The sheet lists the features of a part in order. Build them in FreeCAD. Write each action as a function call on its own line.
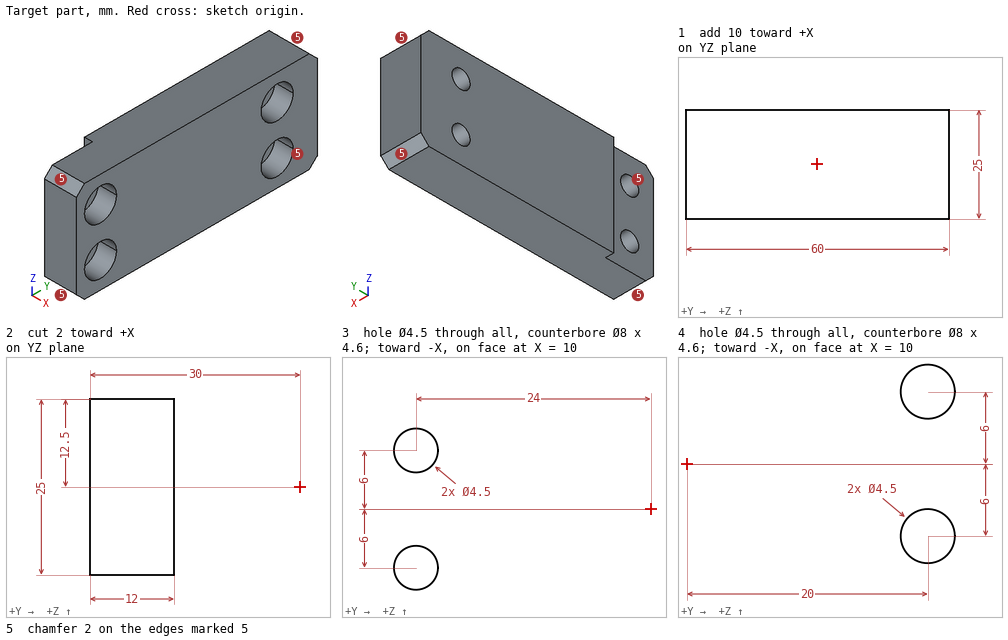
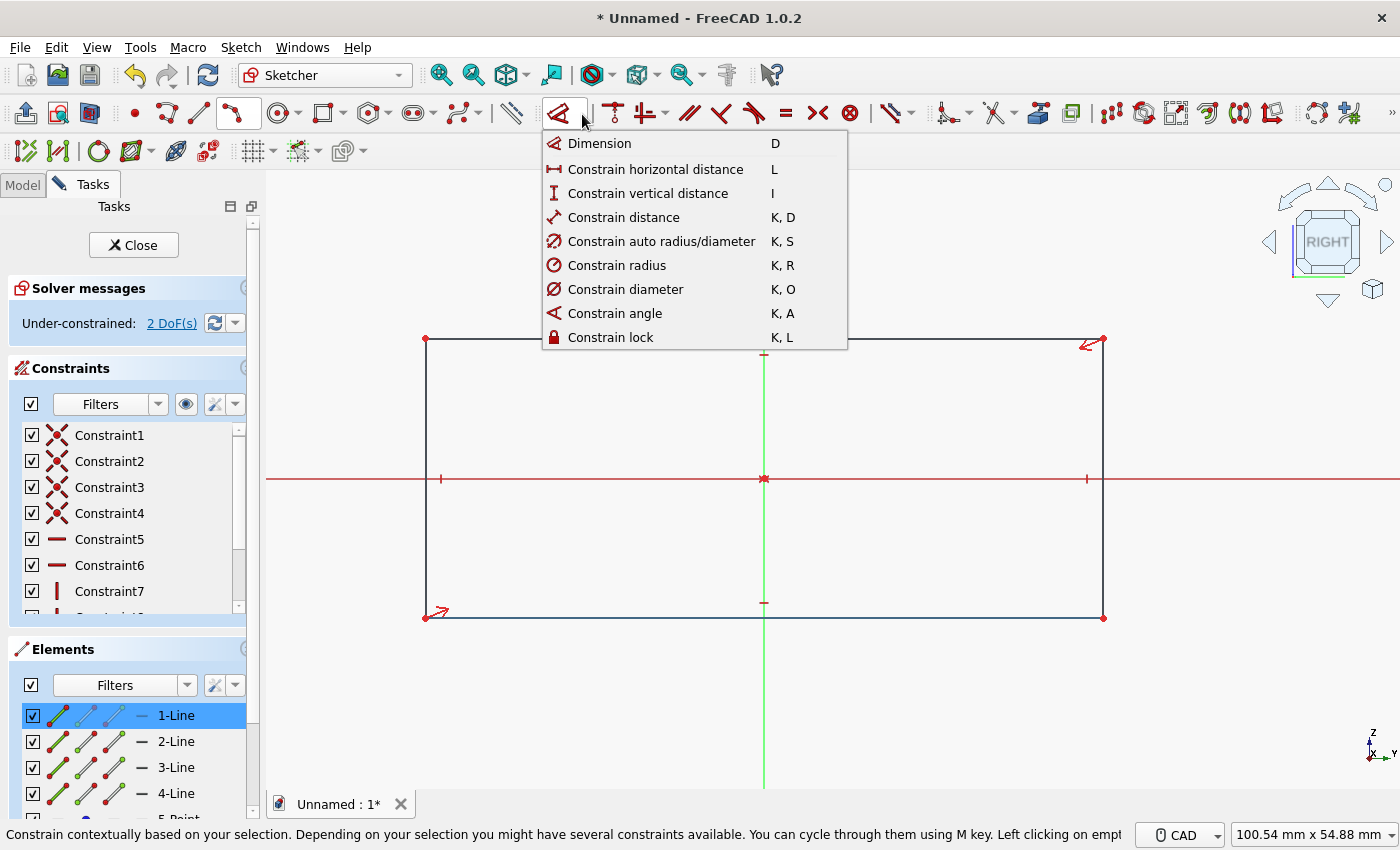
click(695, 169)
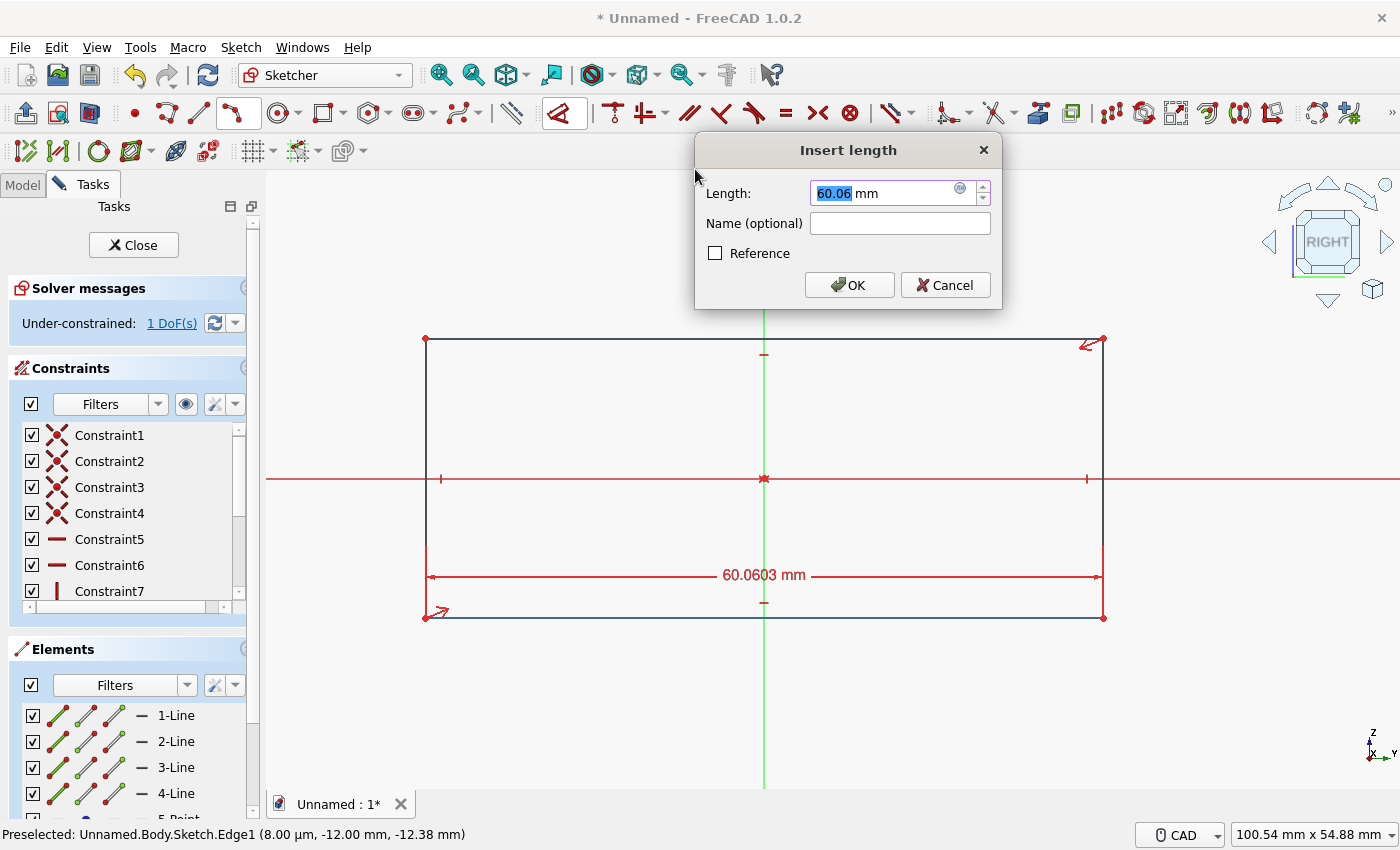
text(60)
key(Return)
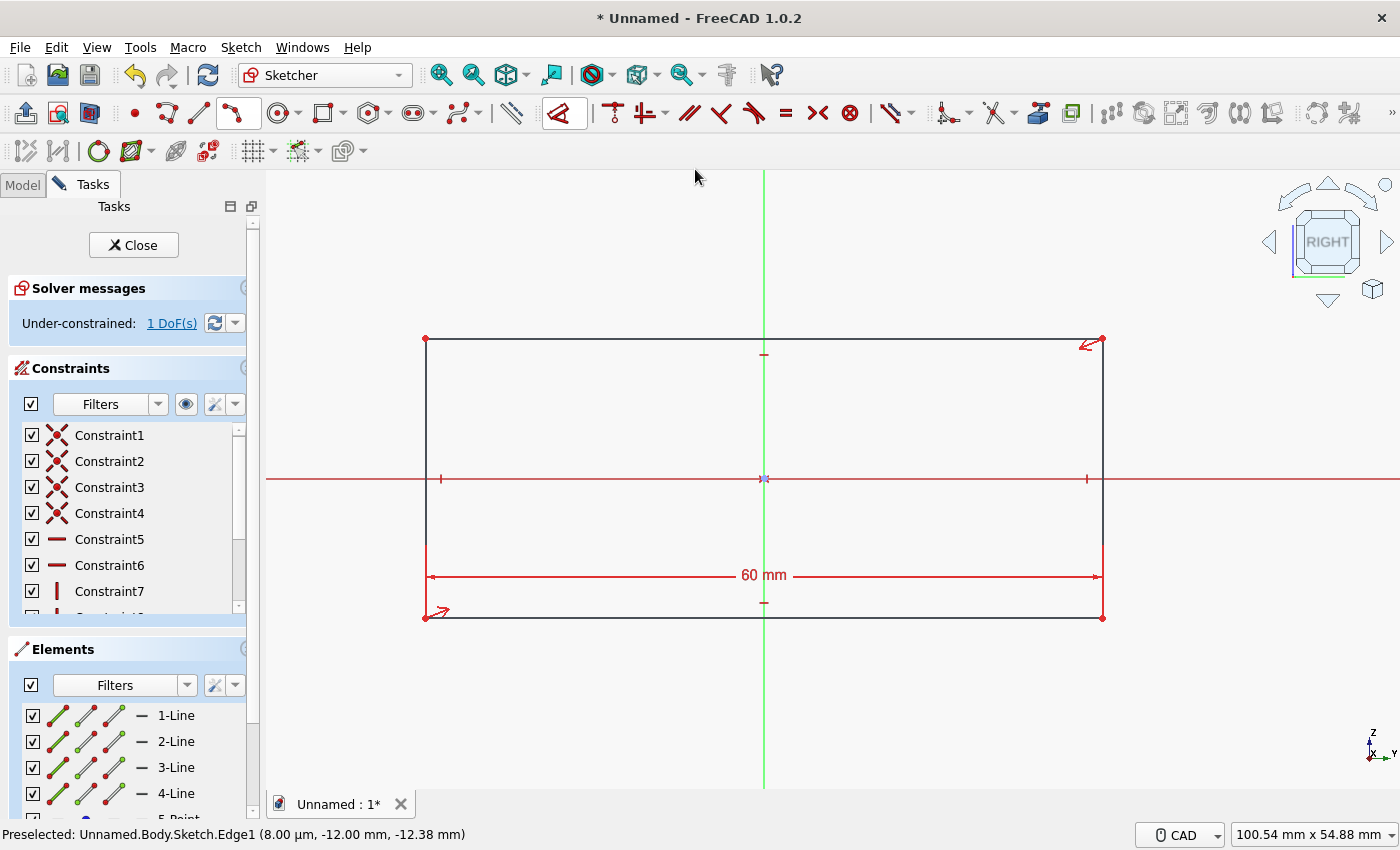
click(1103, 535)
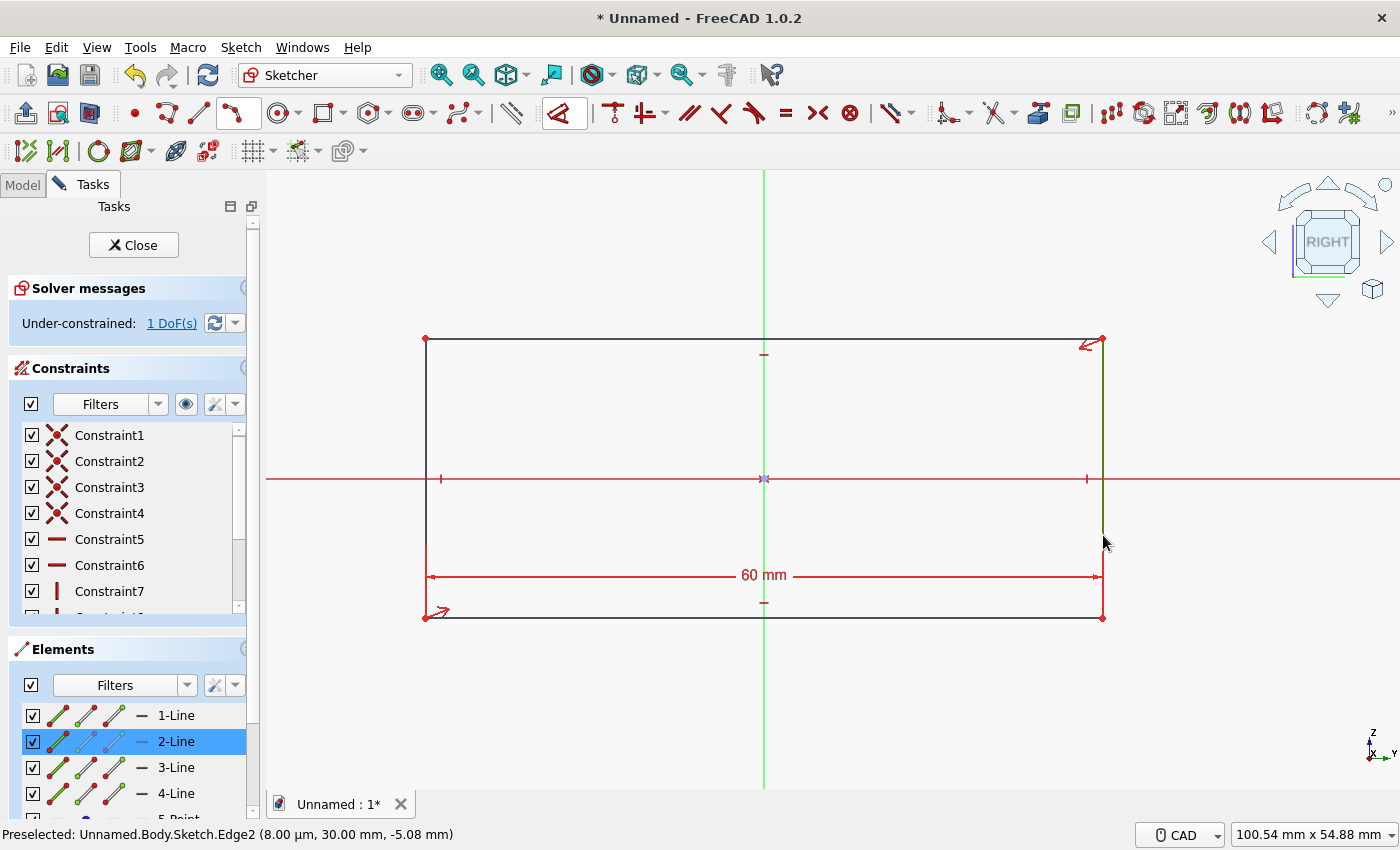
key(i)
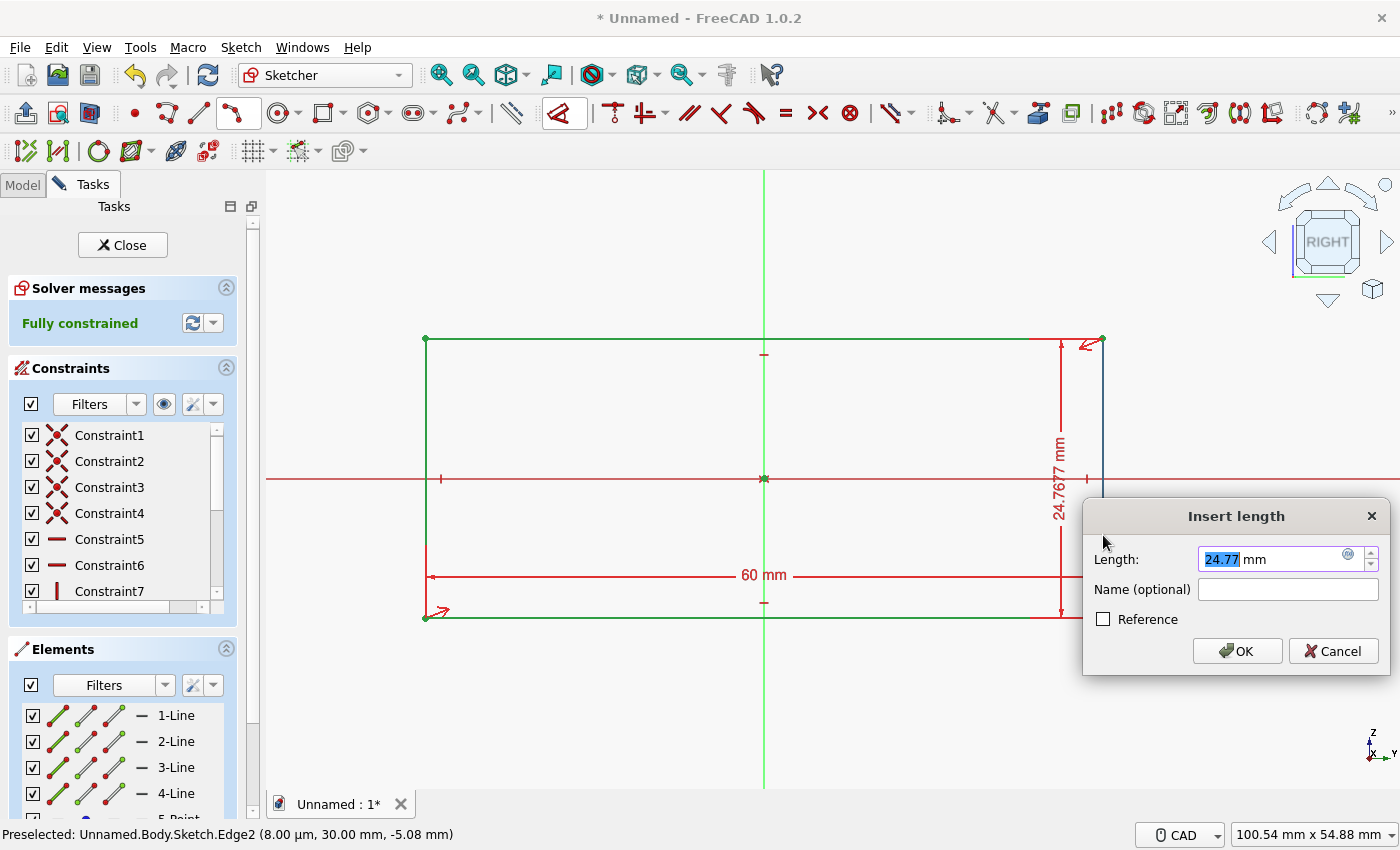
text(25)
key(Return)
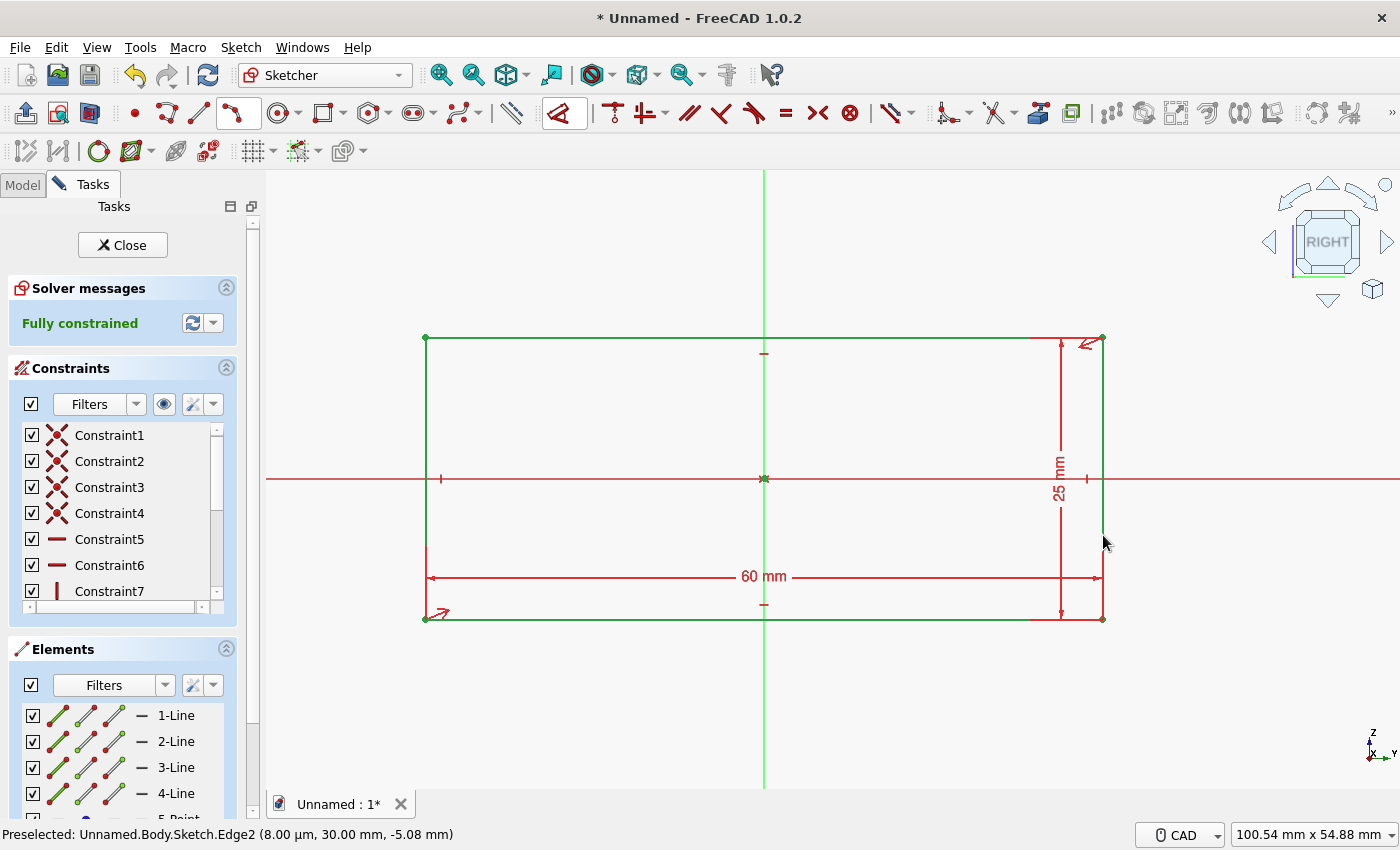
click(123, 245)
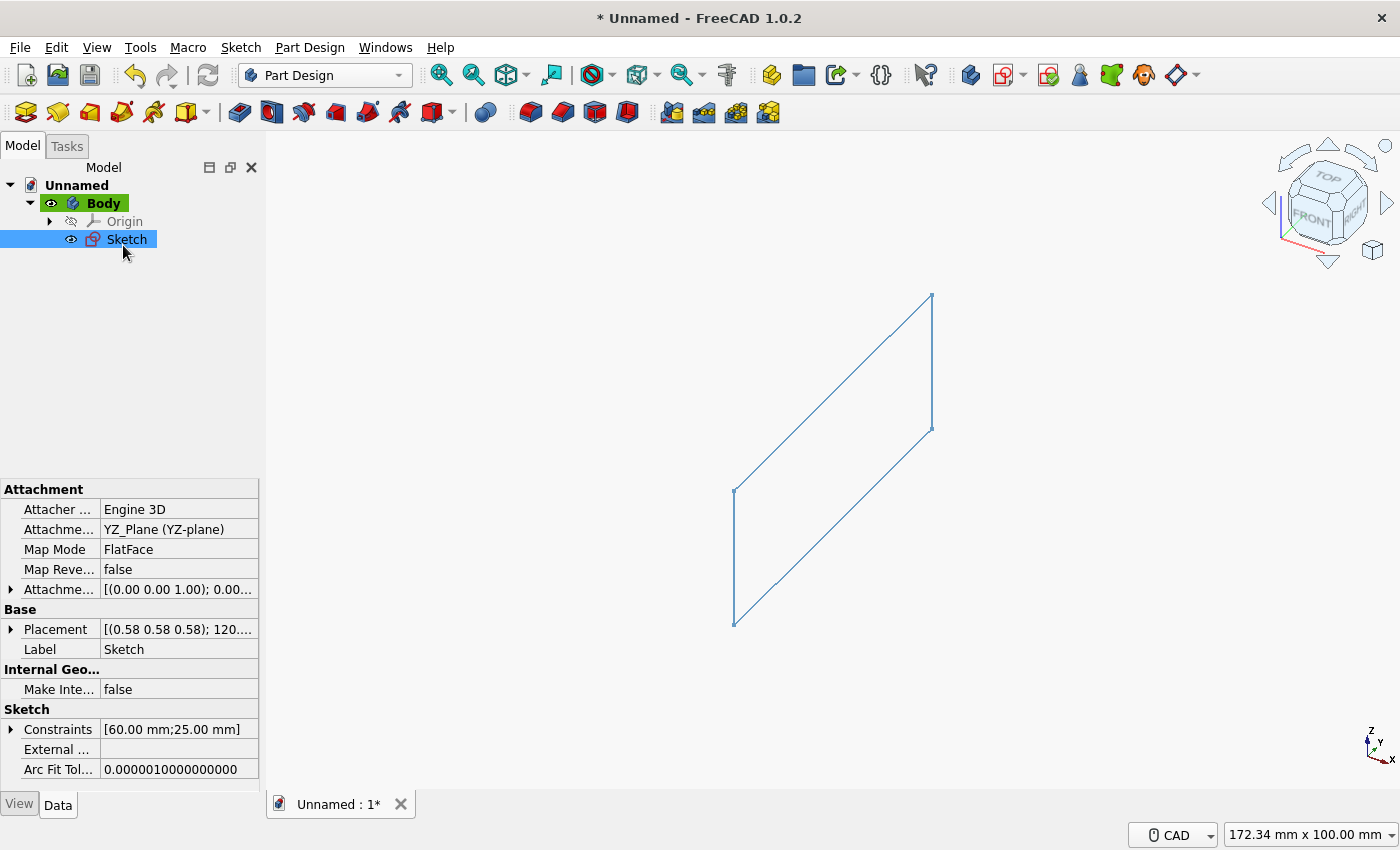
click(26, 112)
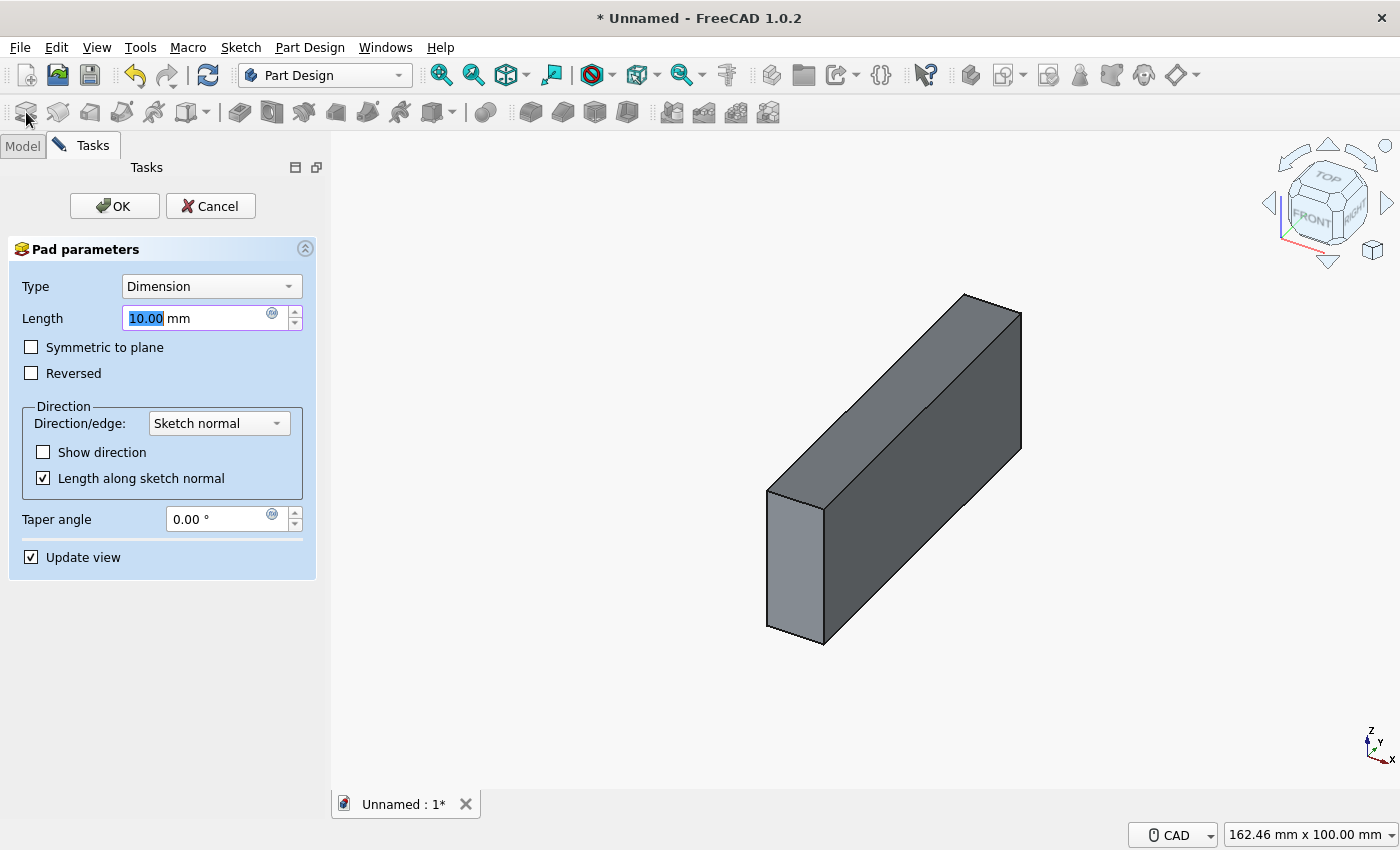
text(10)
key(Tab)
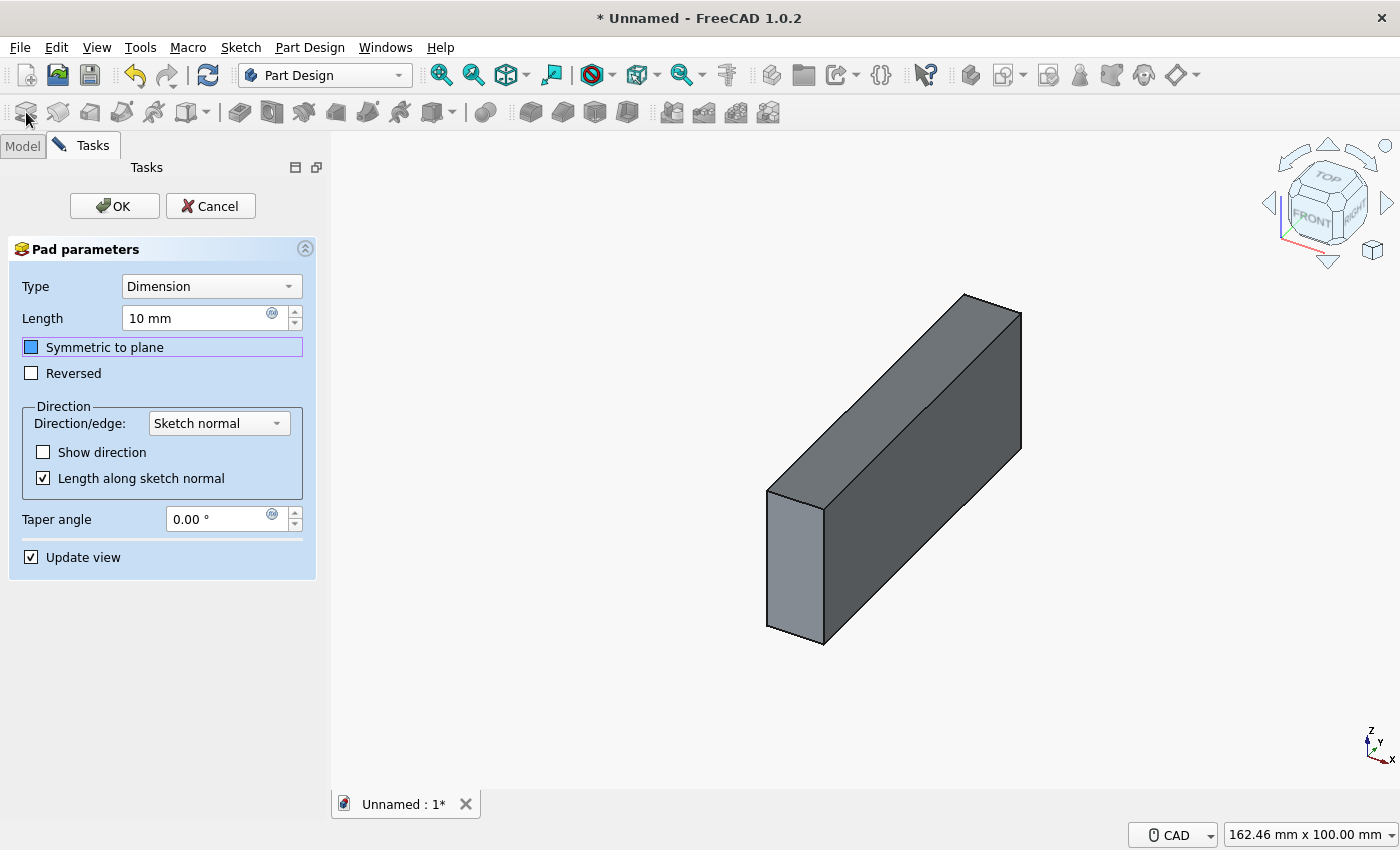
click(115, 206)